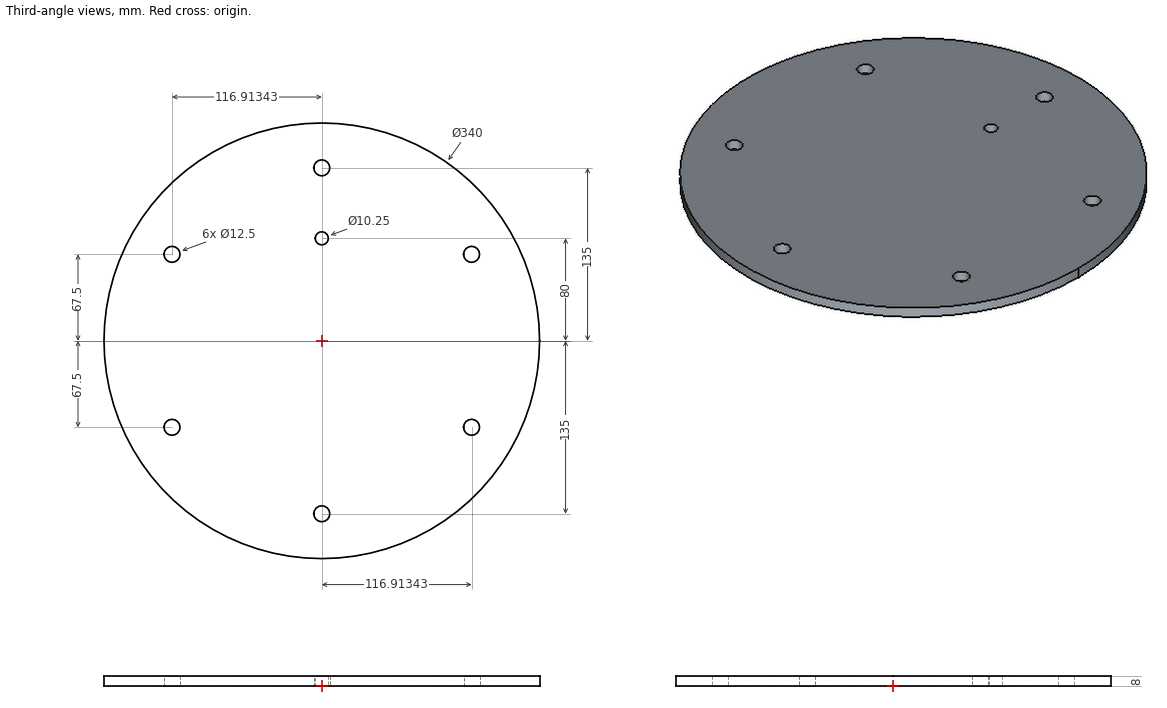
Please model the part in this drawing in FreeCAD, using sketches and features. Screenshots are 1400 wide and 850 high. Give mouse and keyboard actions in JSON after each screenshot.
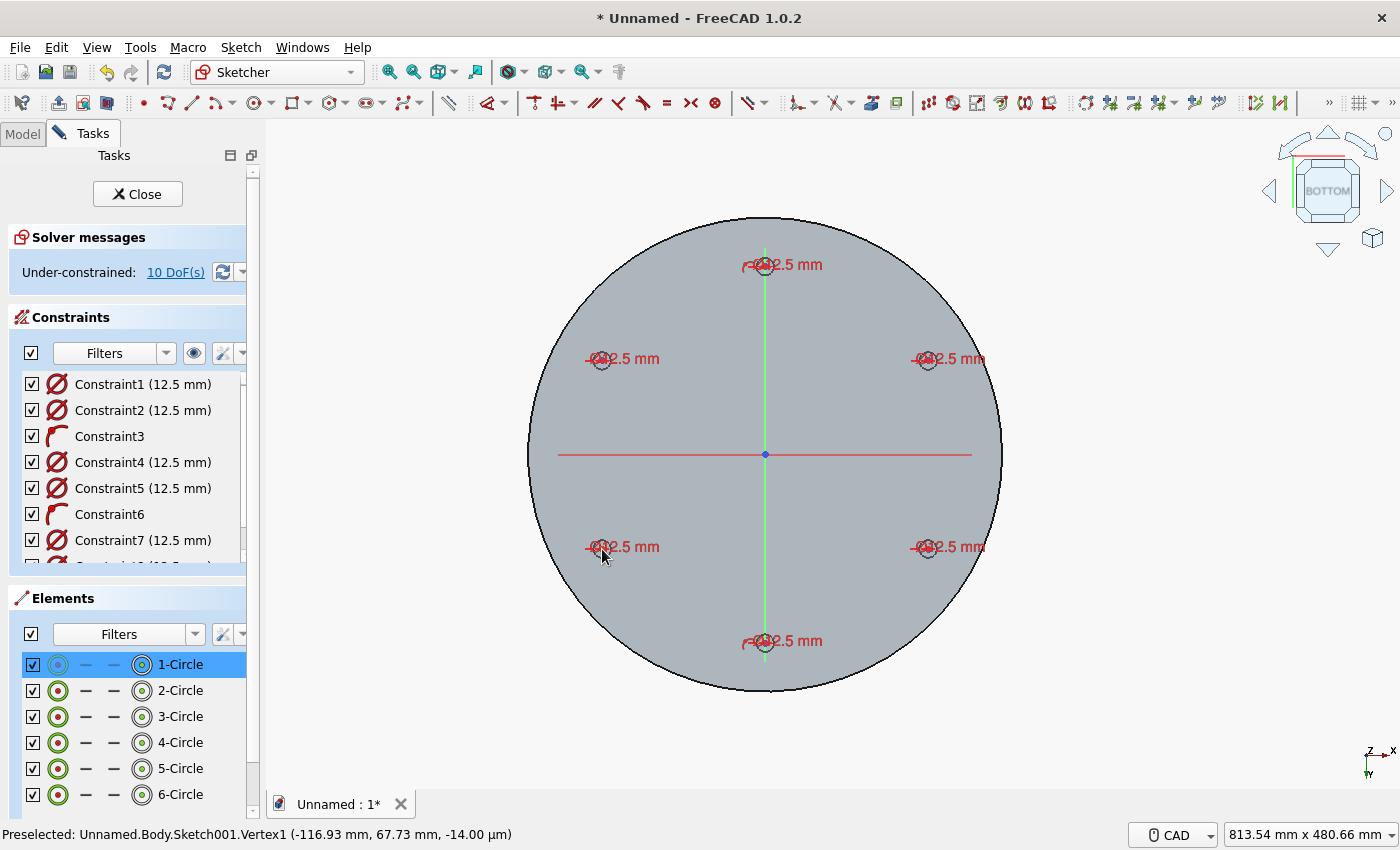
{"action": "left_click", "coordinate": [602, 361]}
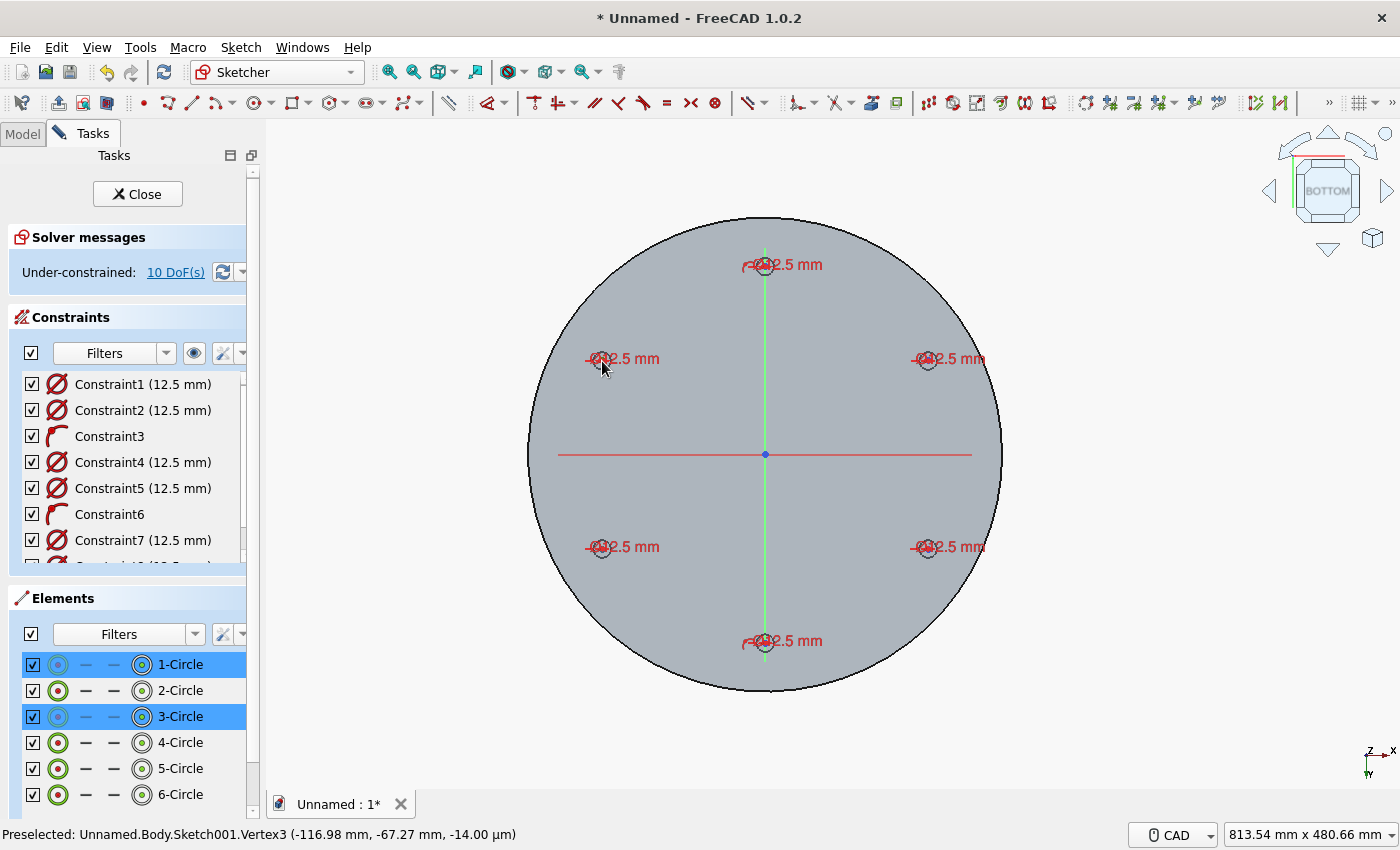
{"action": "left_click", "coordinate": [576, 104]}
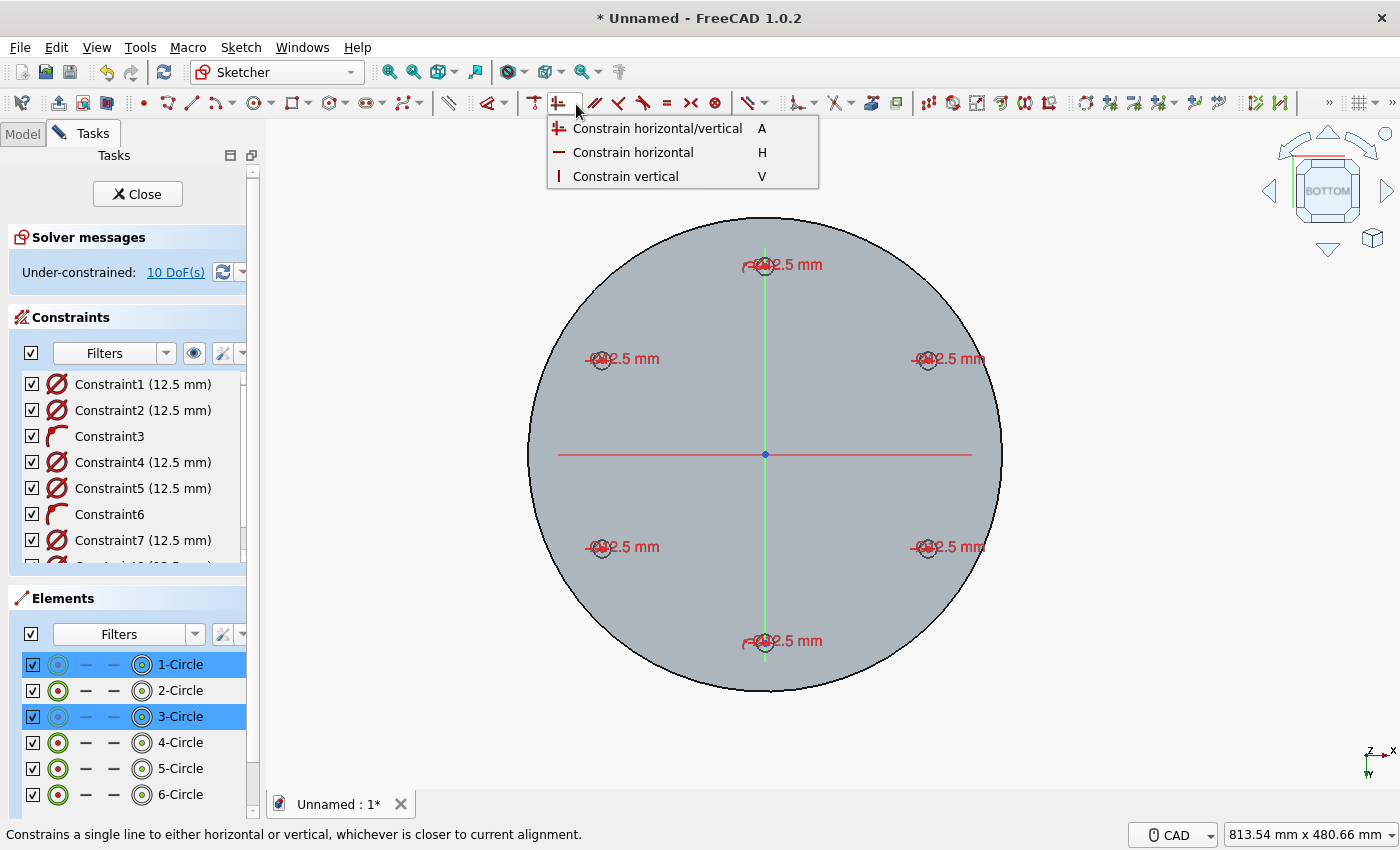
{"action": "left_click", "coordinate": [683, 176]}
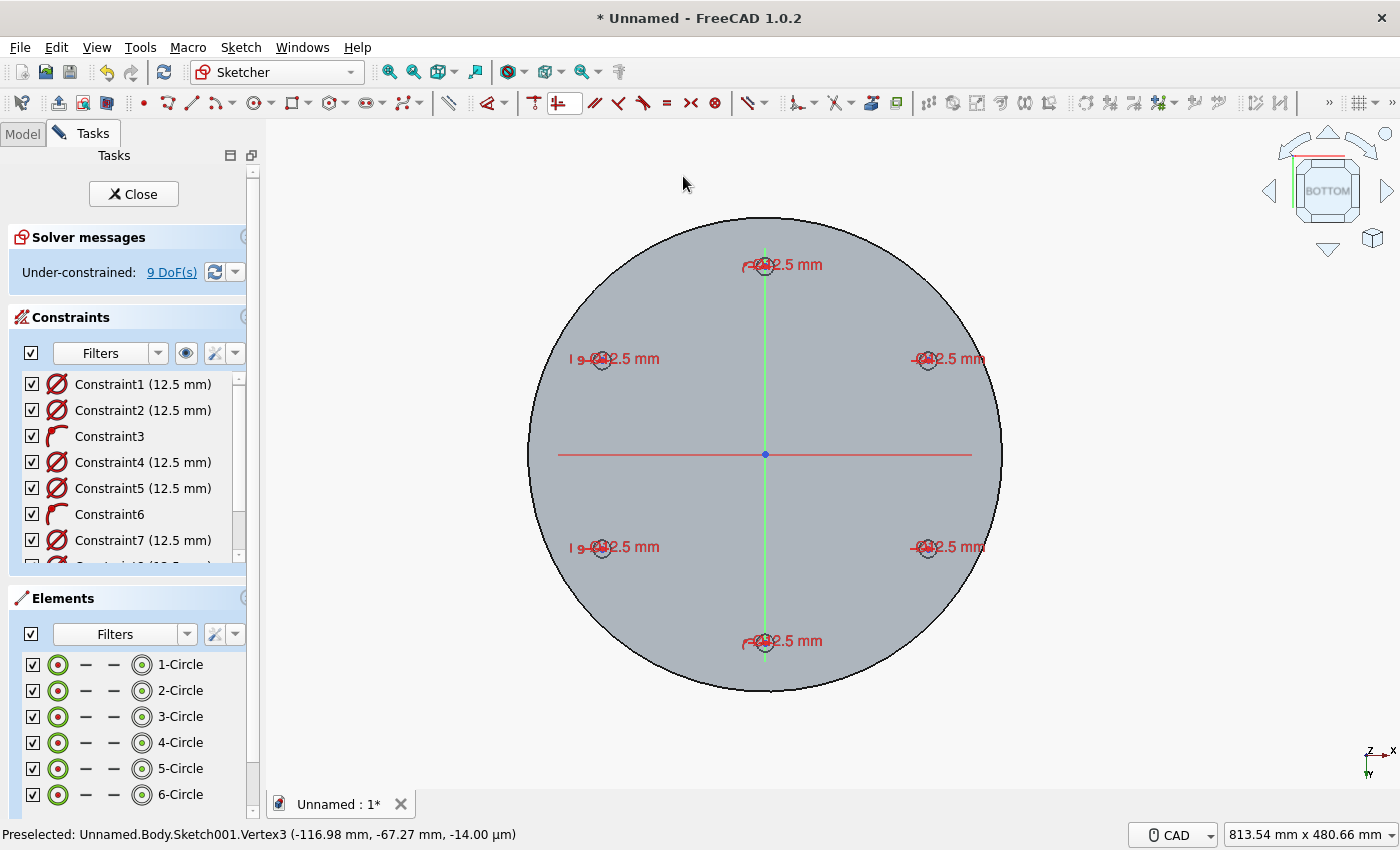
{"action": "left_click", "coordinate": [602, 361]}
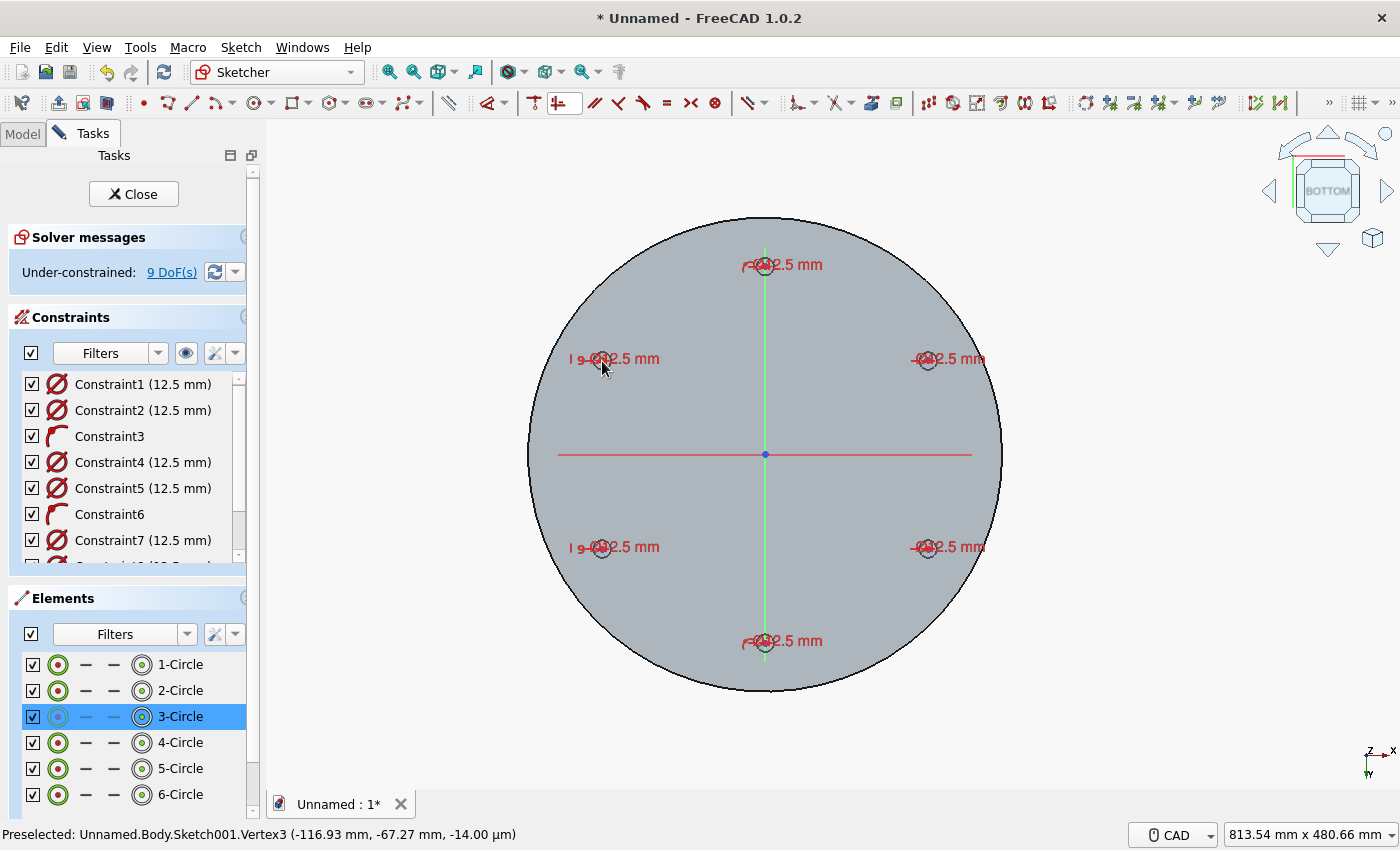
{"action": "left_click", "coordinate": [928, 361]}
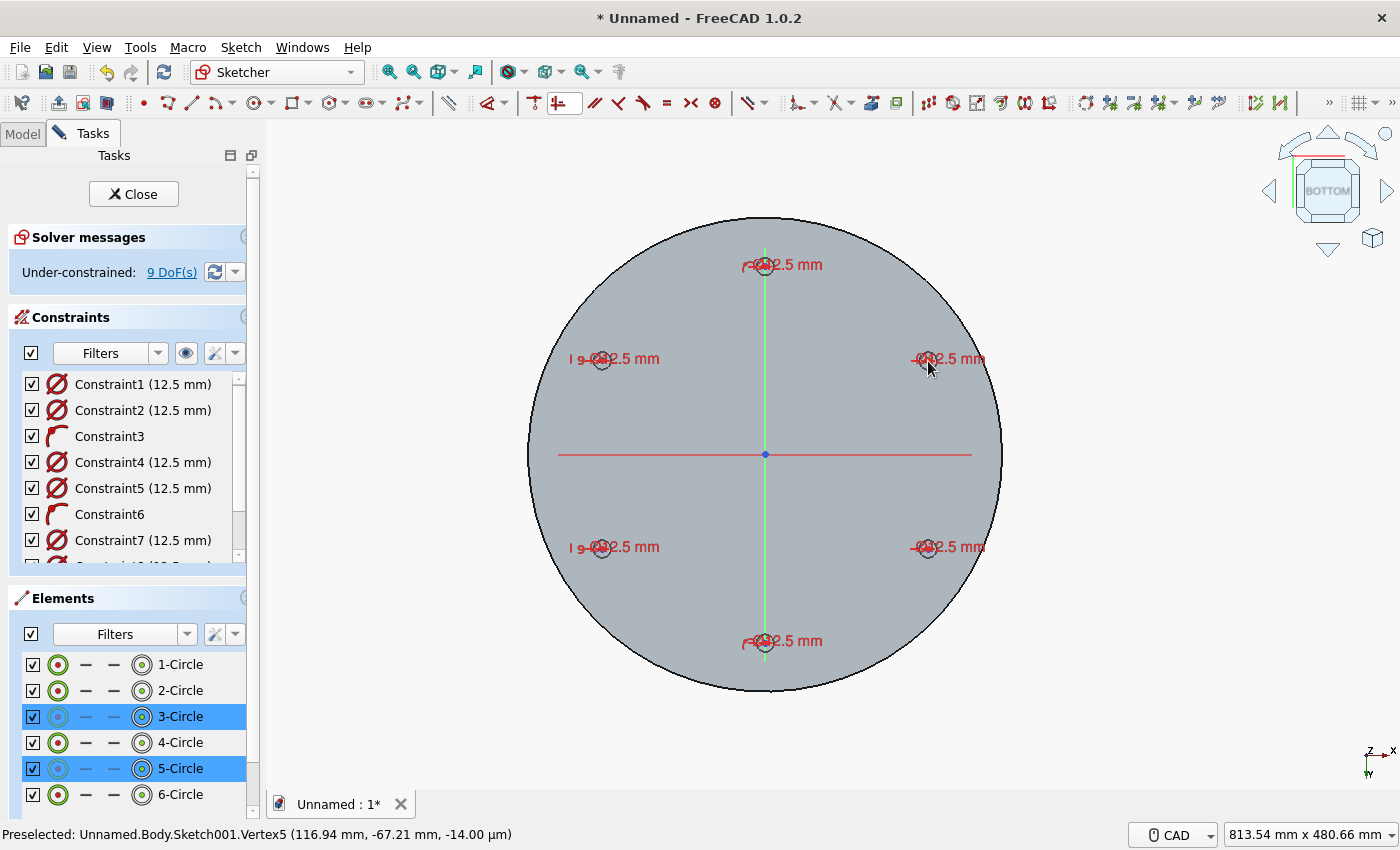
{"action": "left_click", "coordinate": [576, 104]}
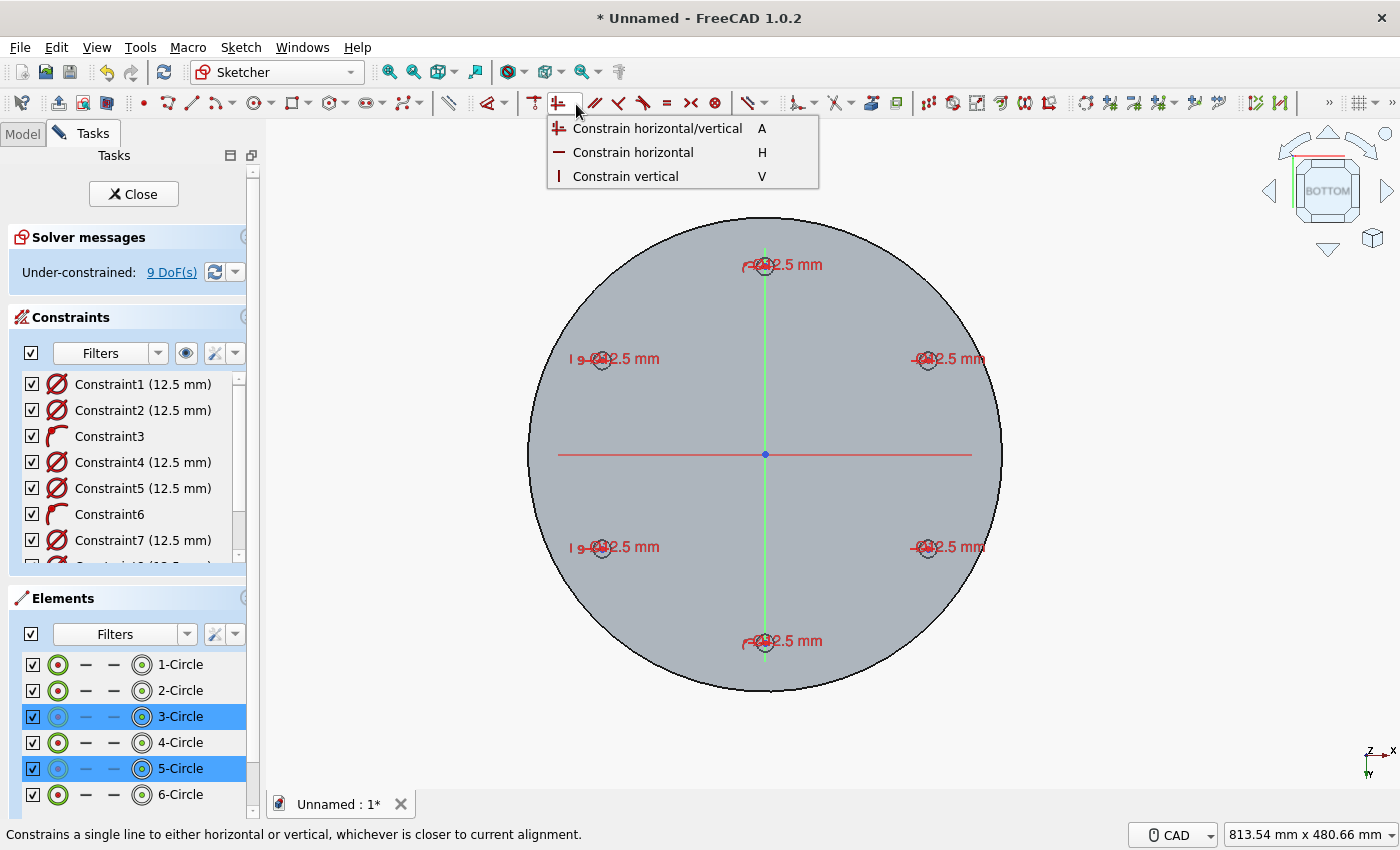
{"action": "left_click", "coordinate": [683, 152]}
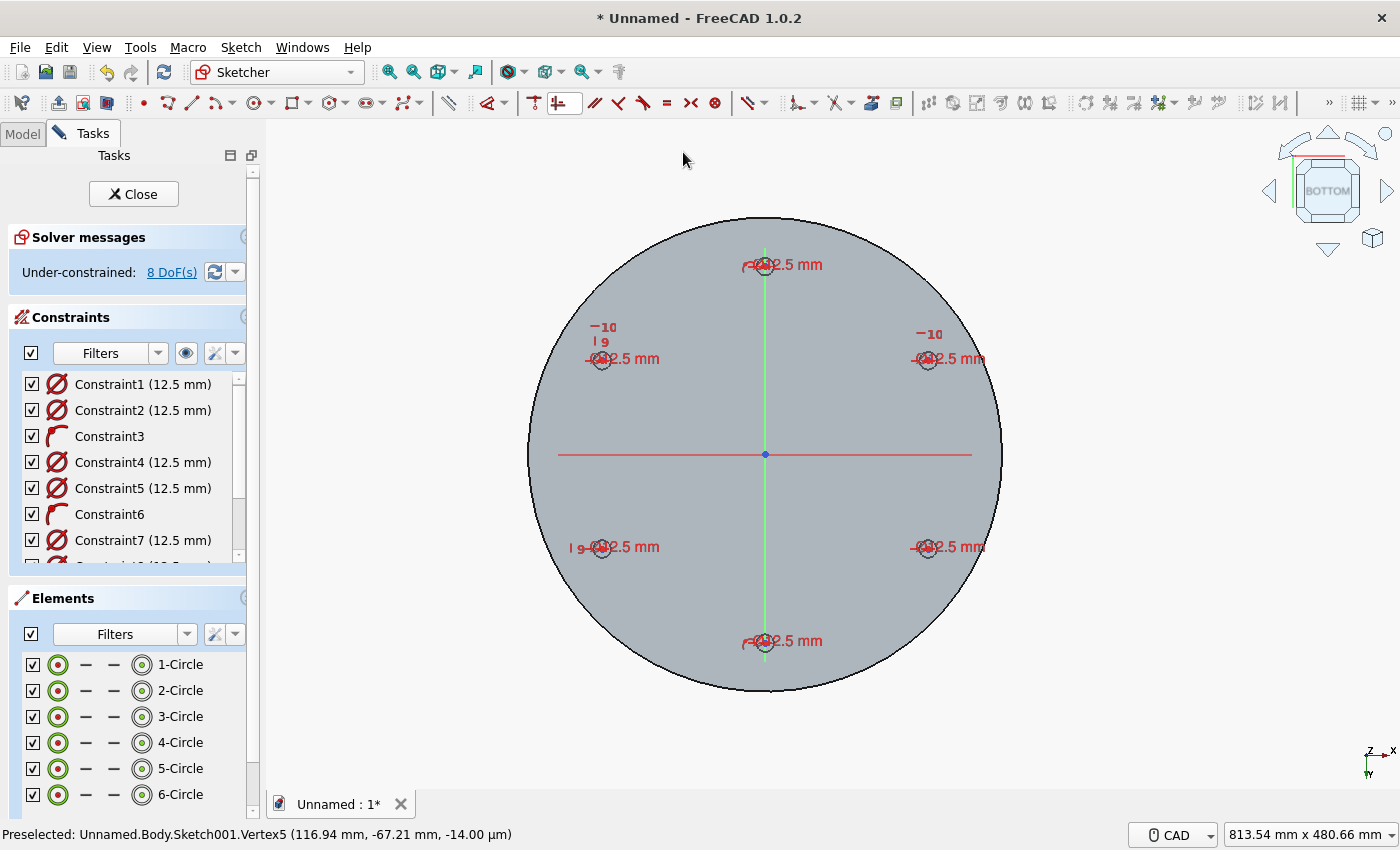
{"action": "left_click", "coordinate": [928, 361]}